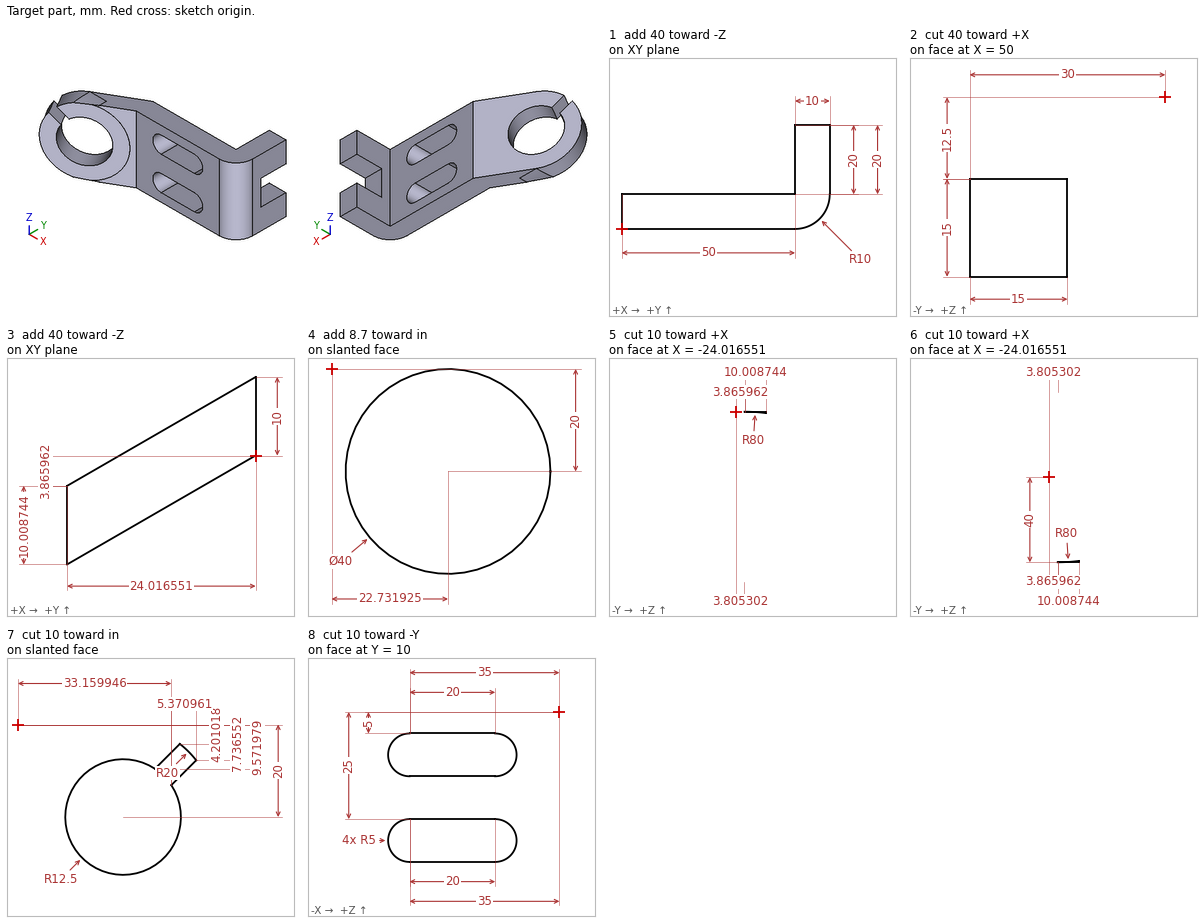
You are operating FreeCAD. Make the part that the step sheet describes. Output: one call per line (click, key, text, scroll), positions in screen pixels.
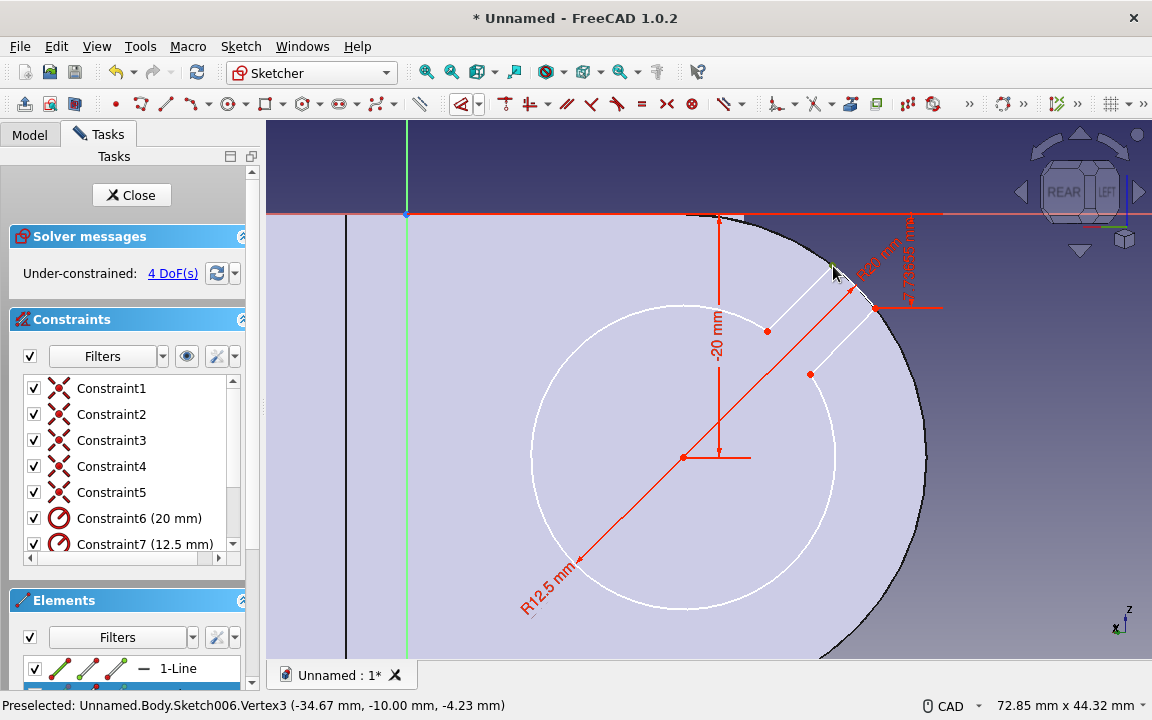
key(i)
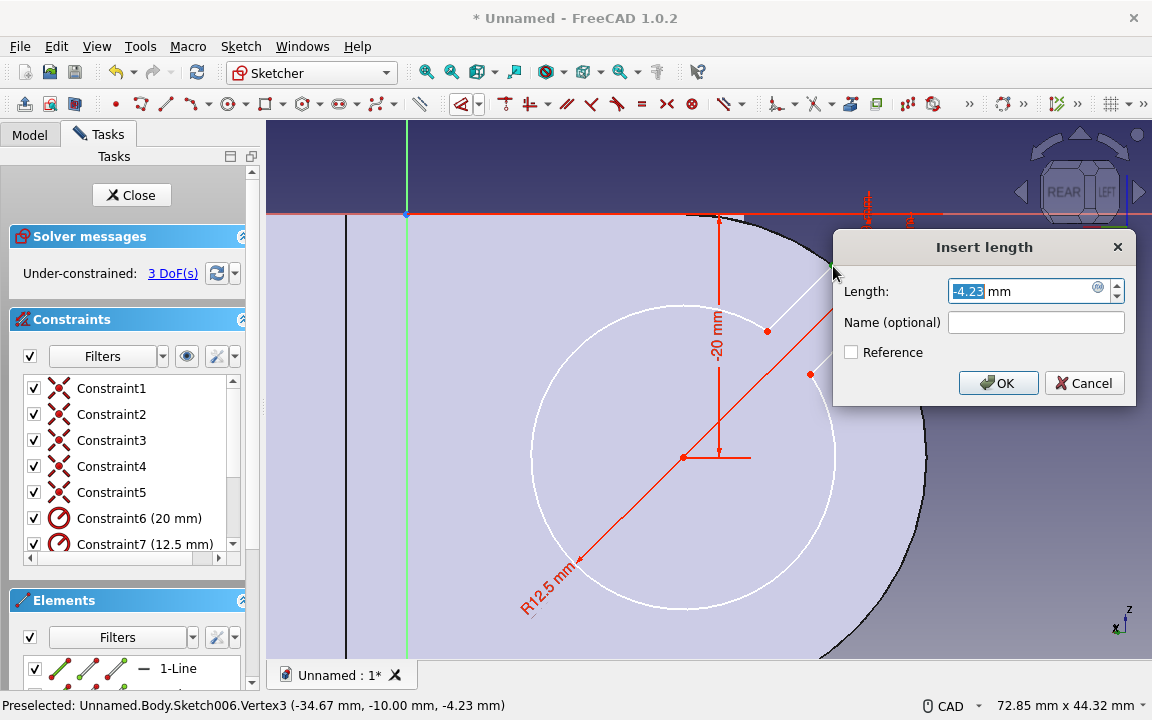
text(-4.201018)
key(Return)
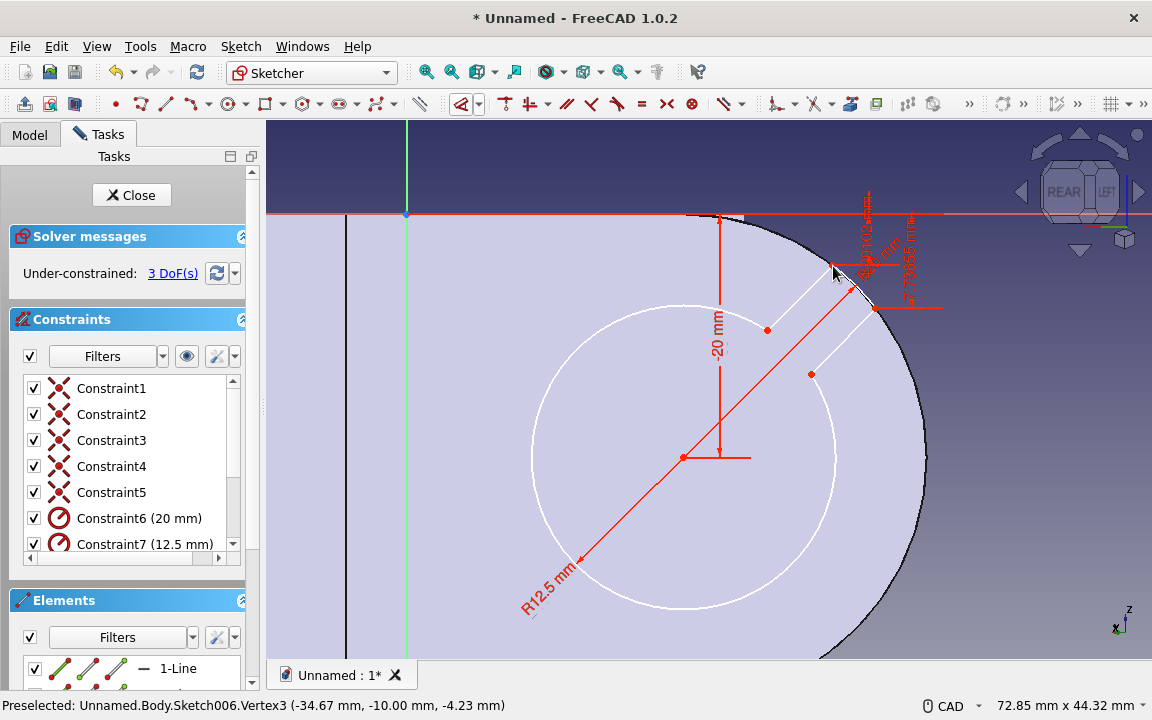
click(768, 331)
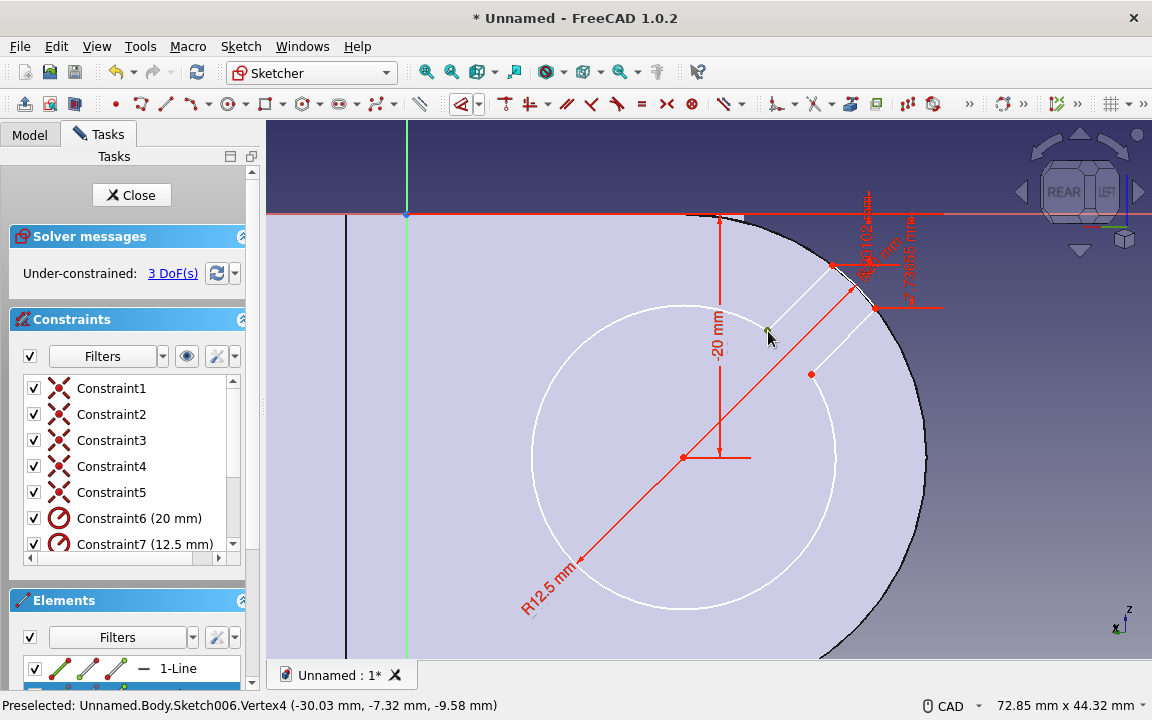
click(478, 104)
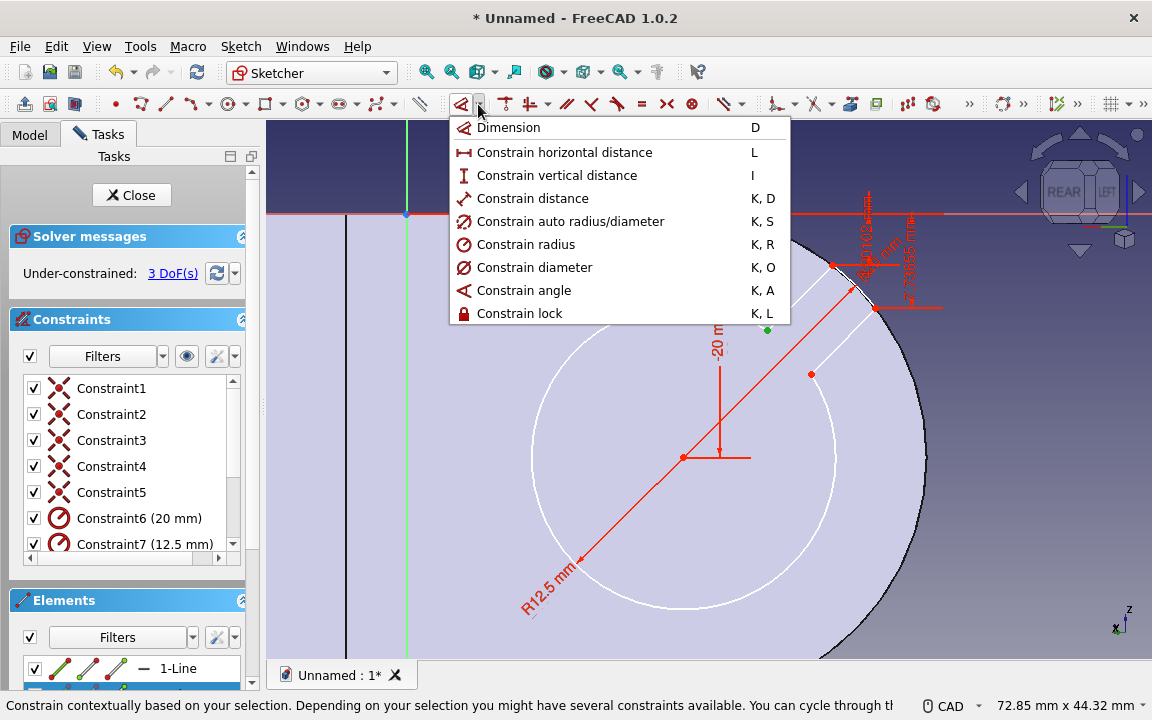
click(620, 176)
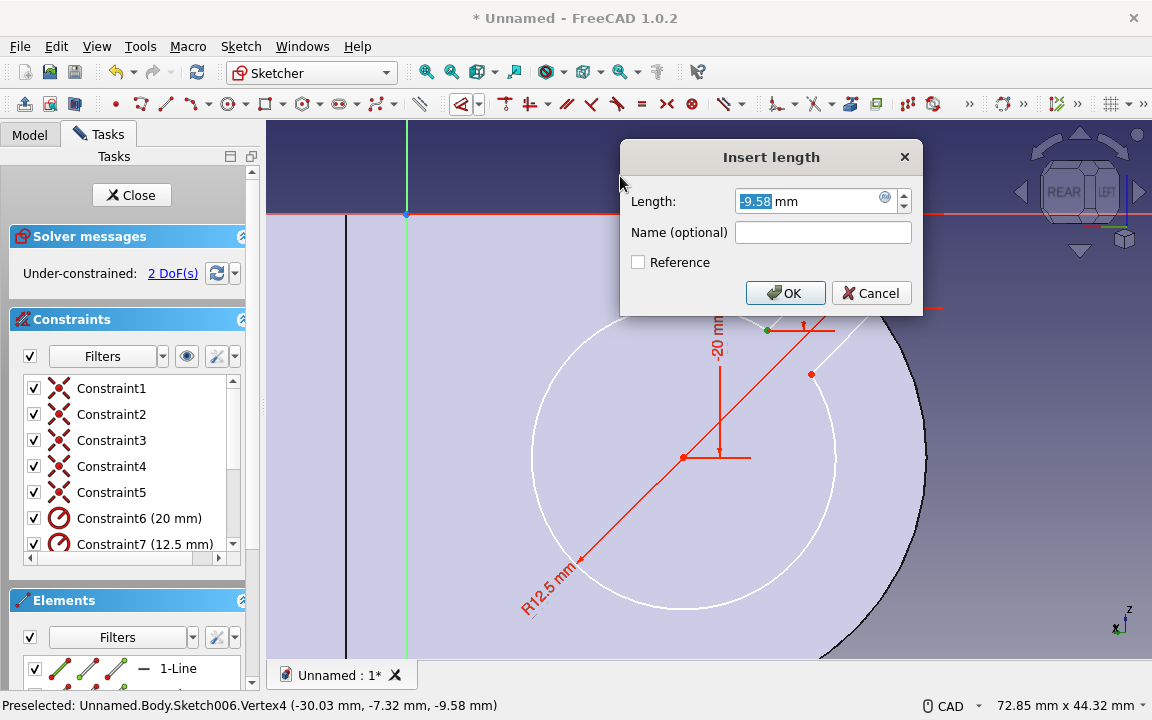
text(-9.571979)
key(Return)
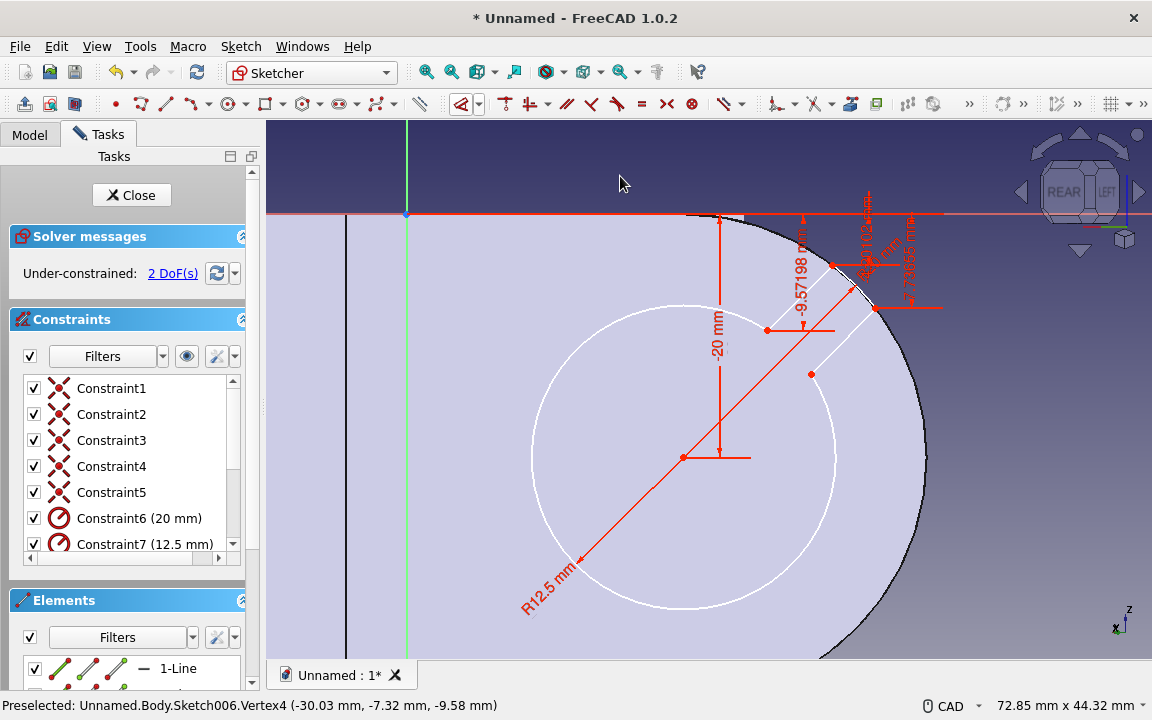
click(831, 355)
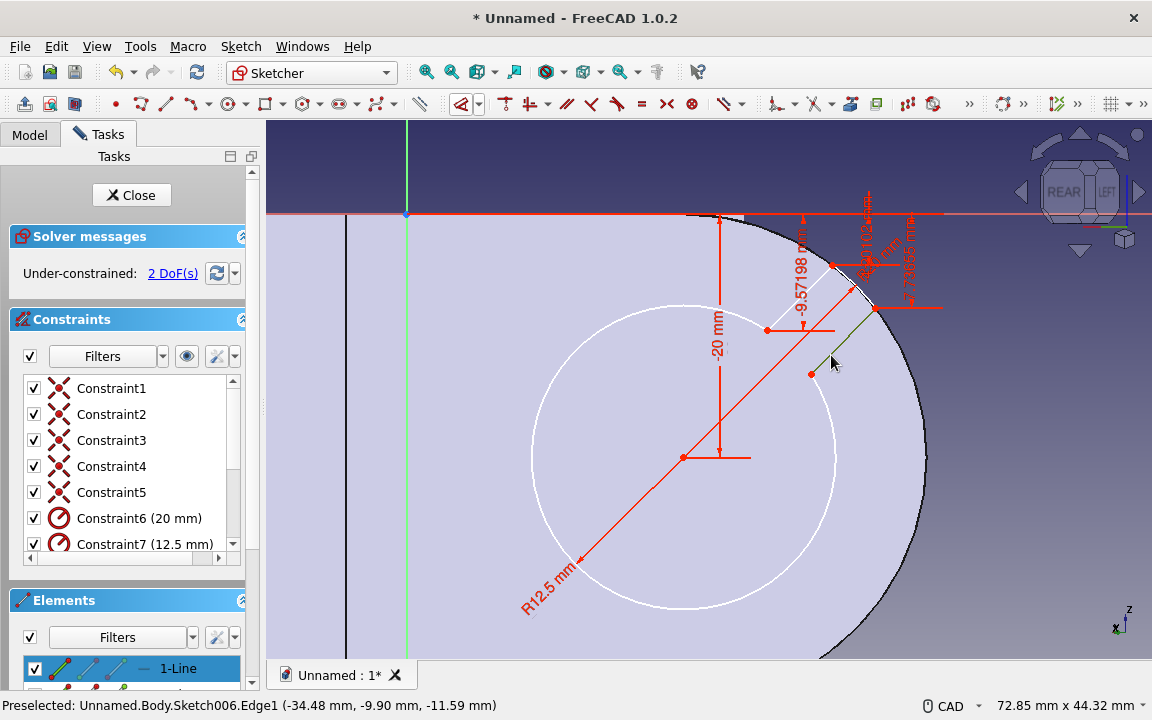
click(478, 104)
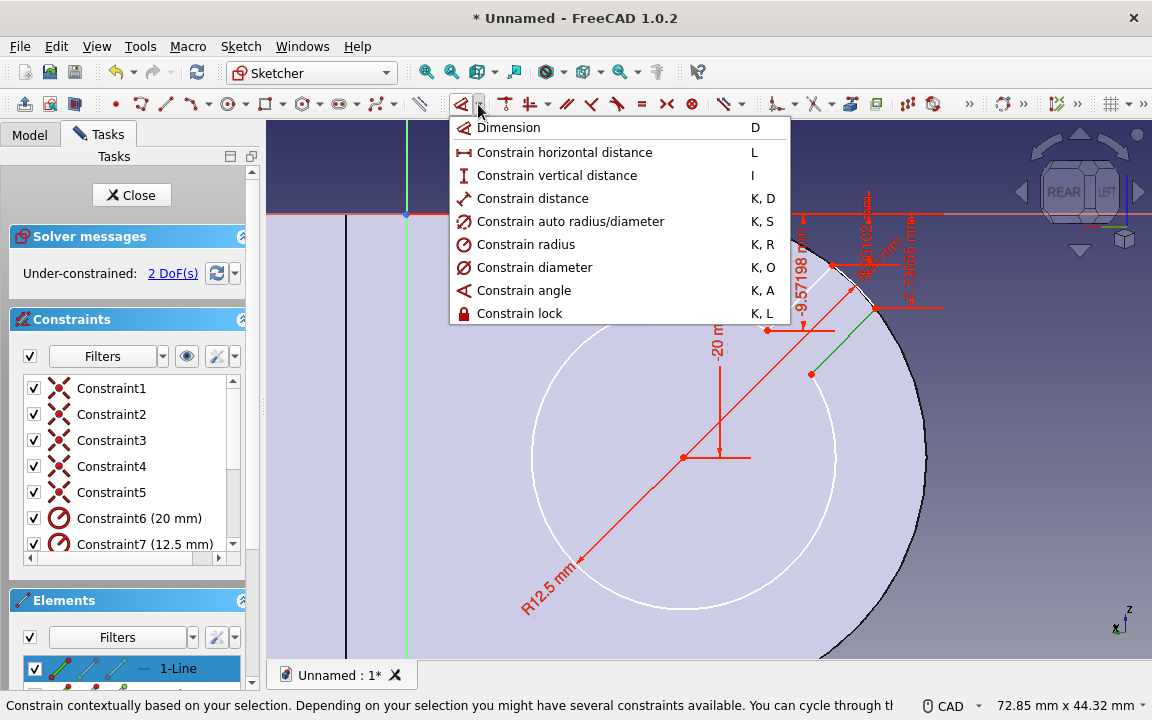
click(620, 152)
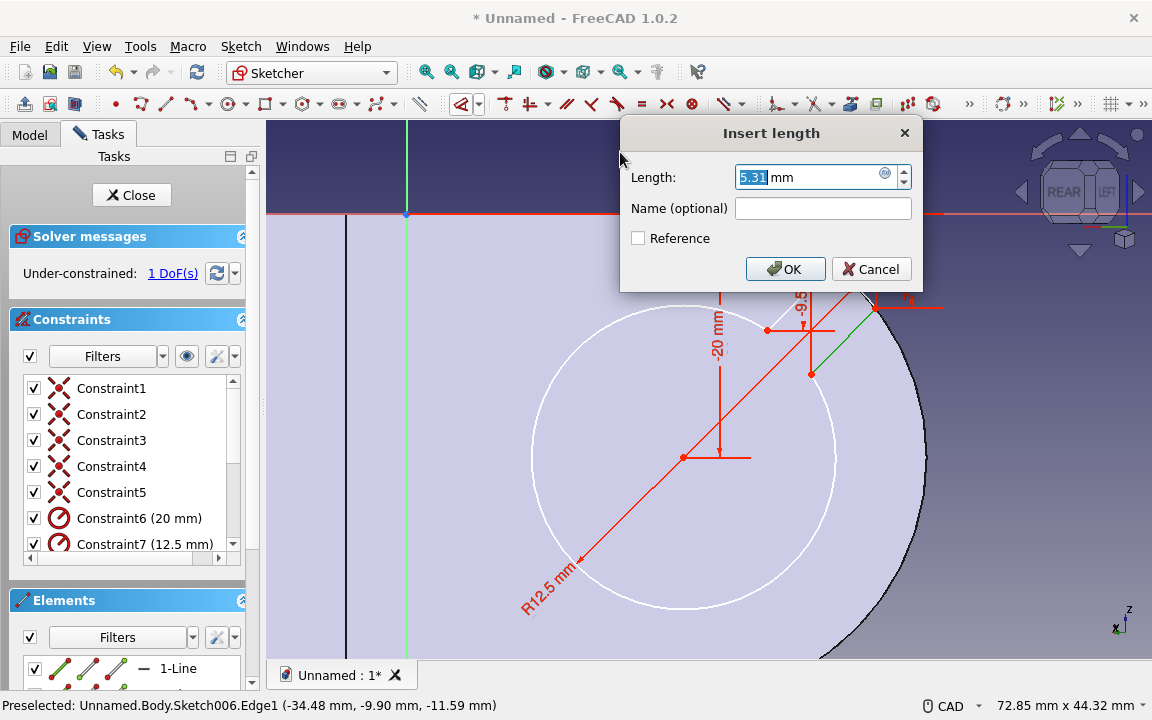
text(5.370961)
key(Return)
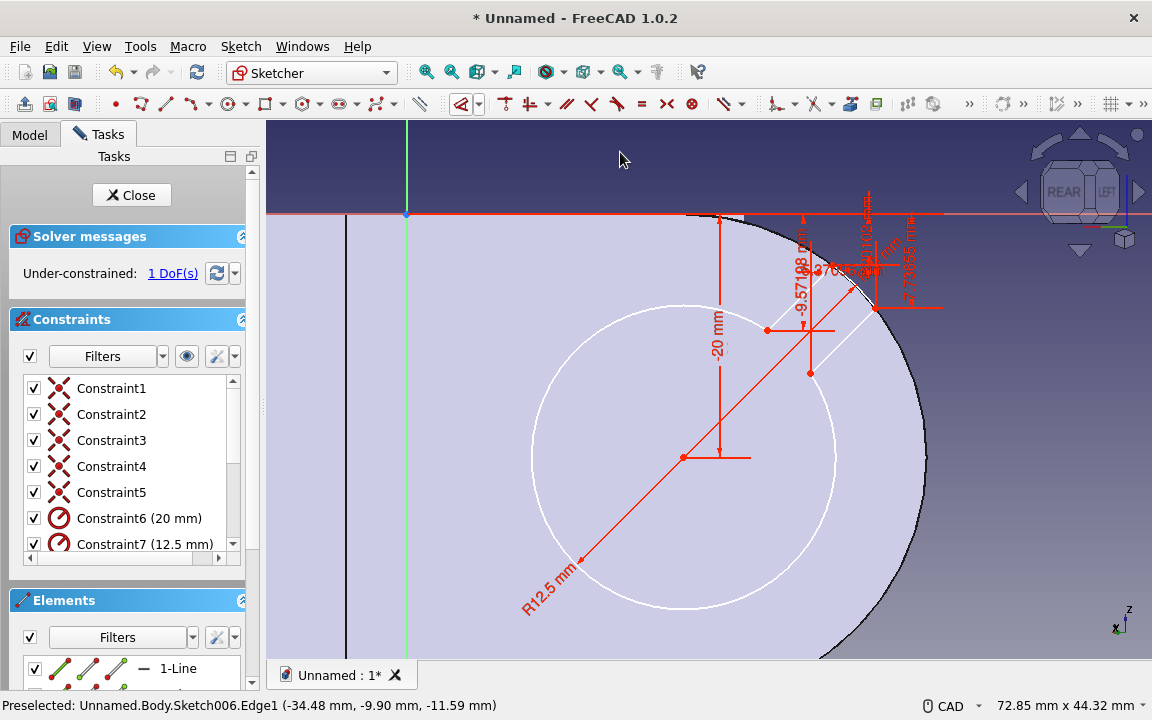
click(811, 374)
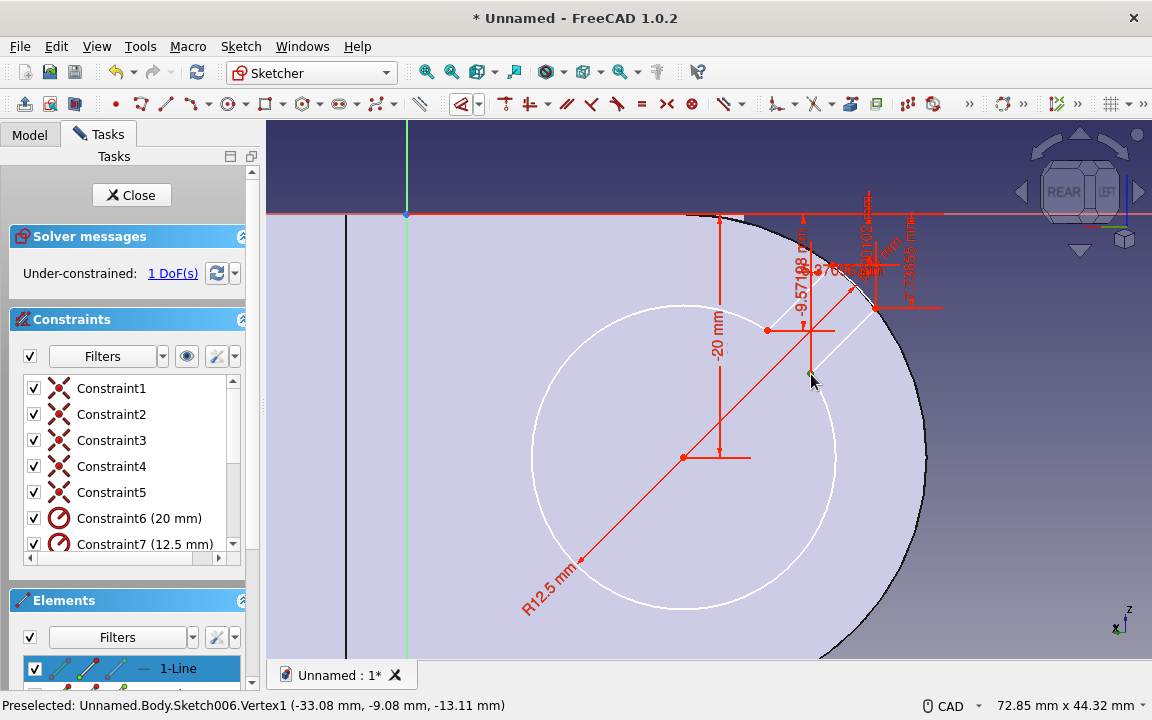
click(478, 104)